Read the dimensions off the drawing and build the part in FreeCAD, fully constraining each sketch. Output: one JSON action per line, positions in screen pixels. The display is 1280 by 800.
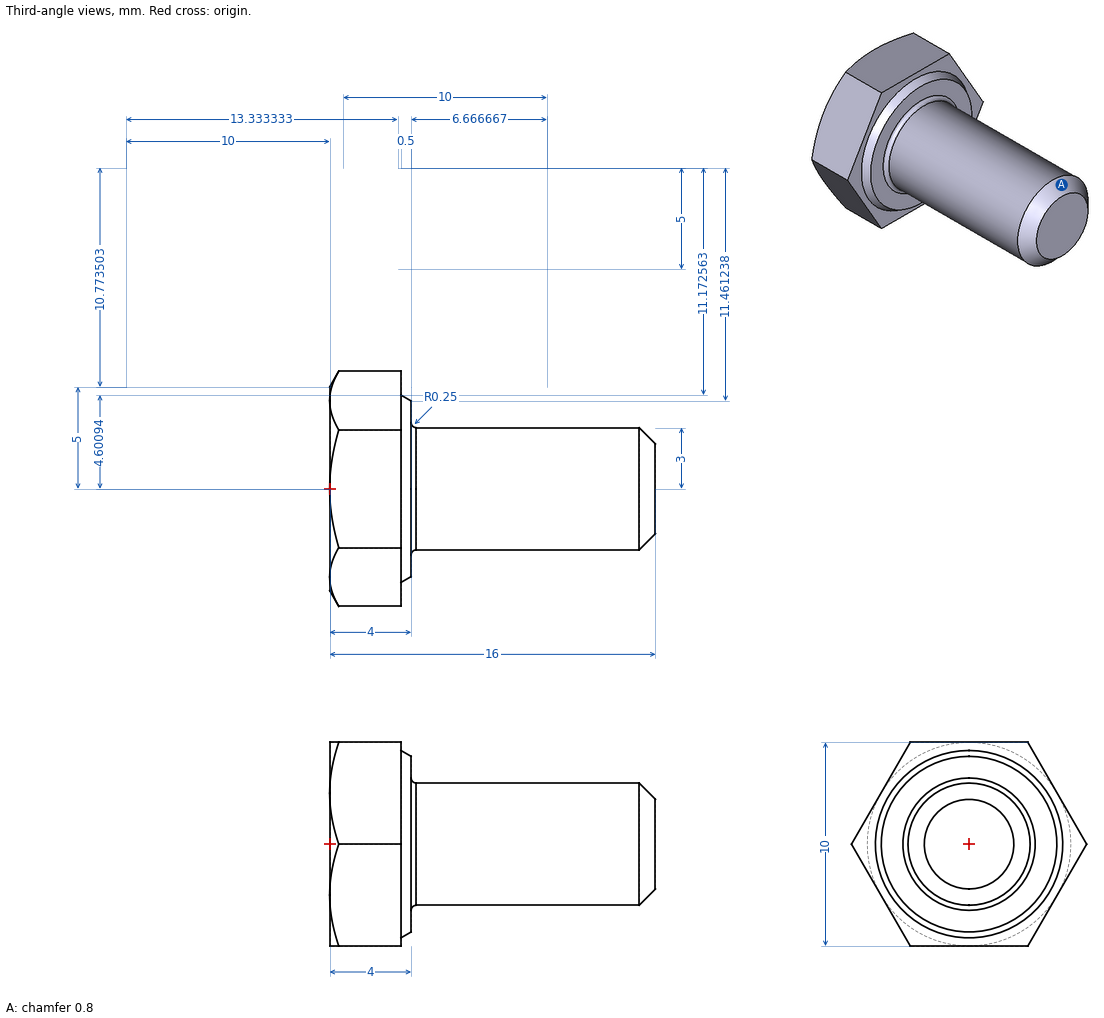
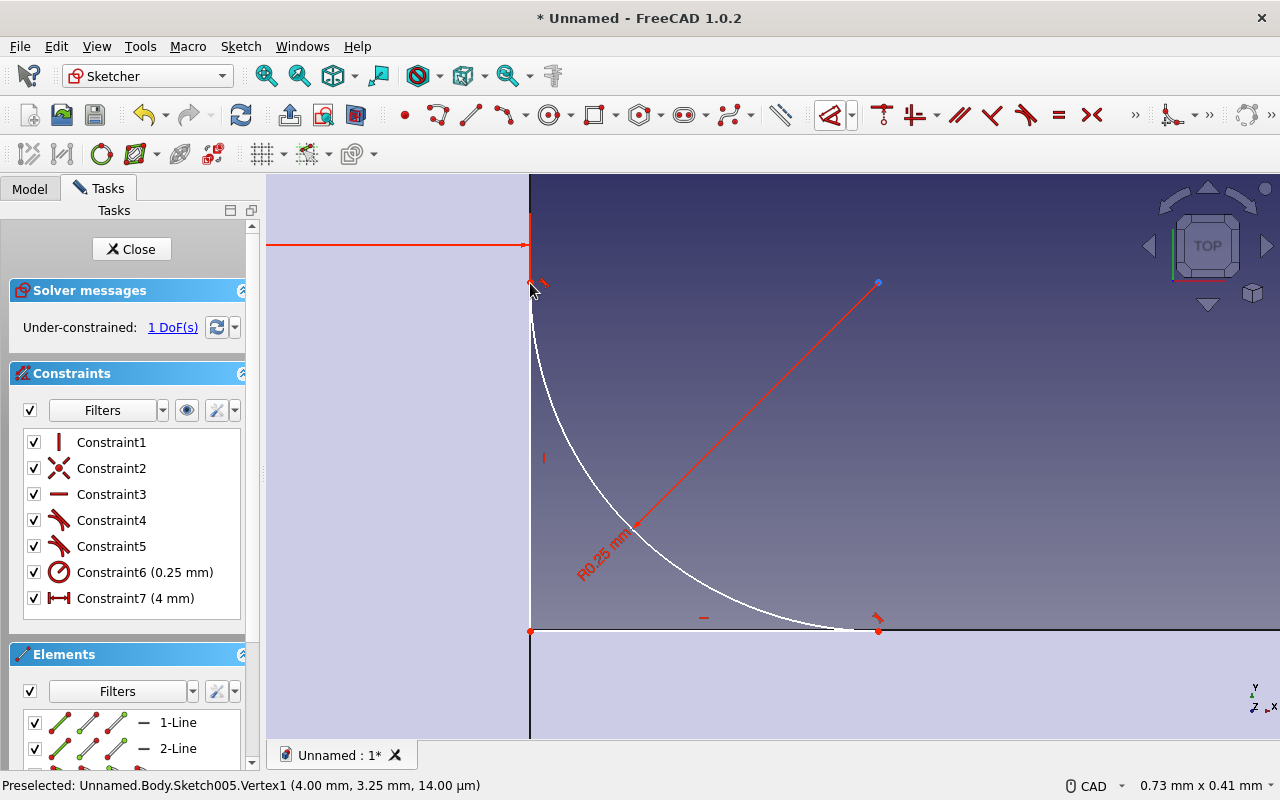
{"action": "left_click", "coordinate": [530, 631]}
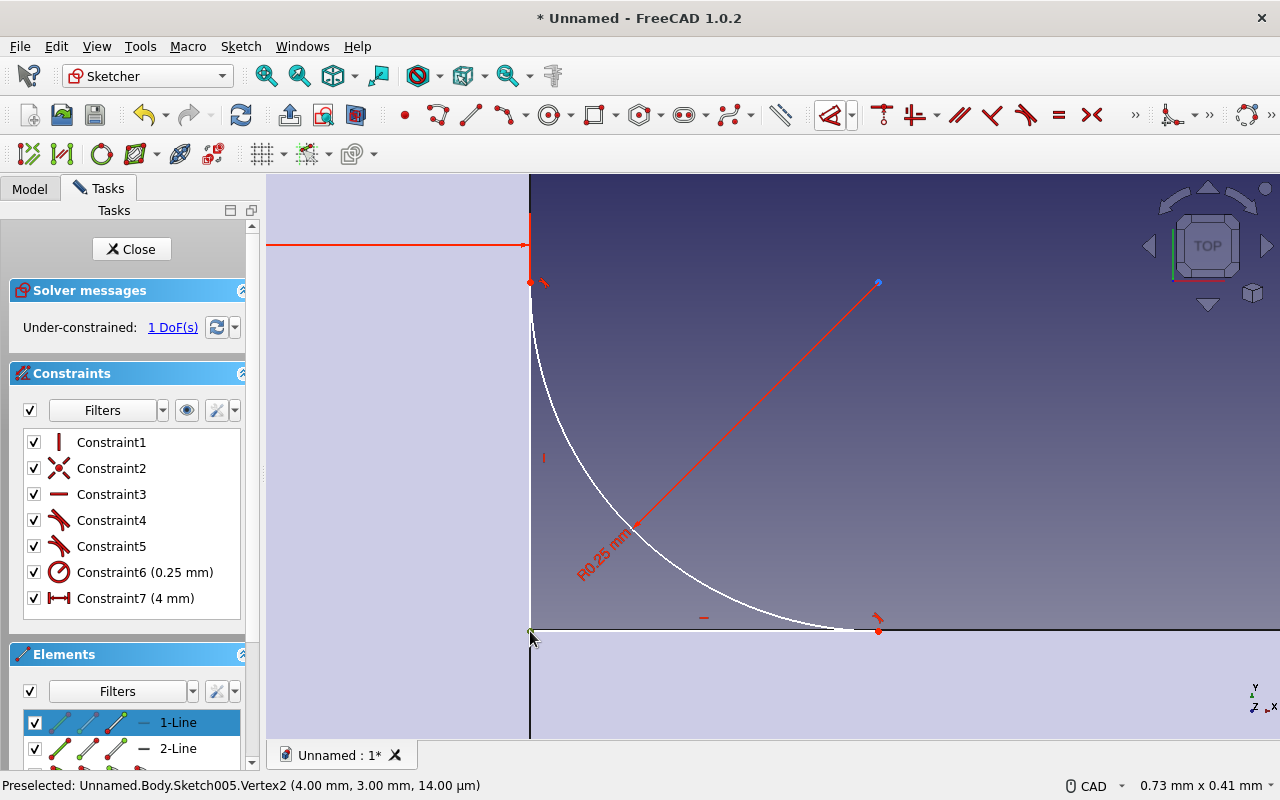
{"action": "left_click", "coordinate": [852, 116]}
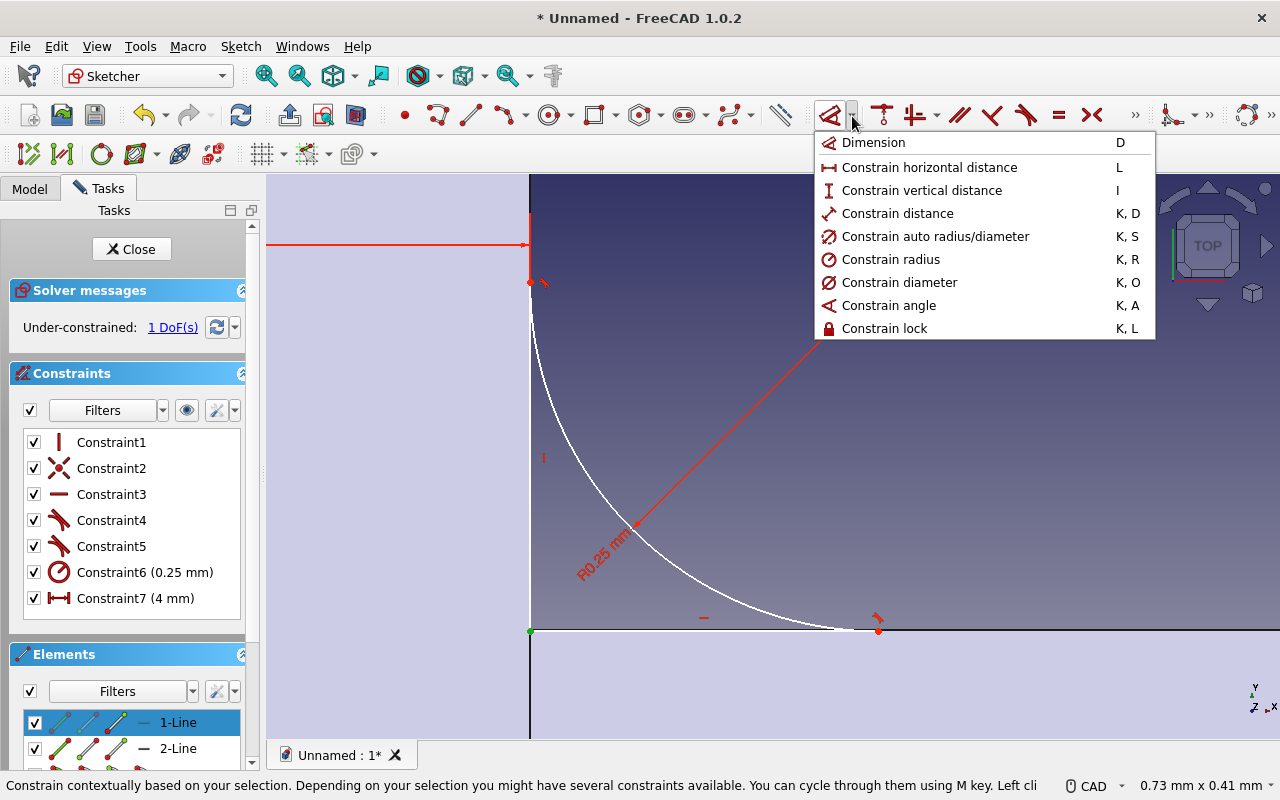
{"action": "left_click", "coordinate": [985, 190]}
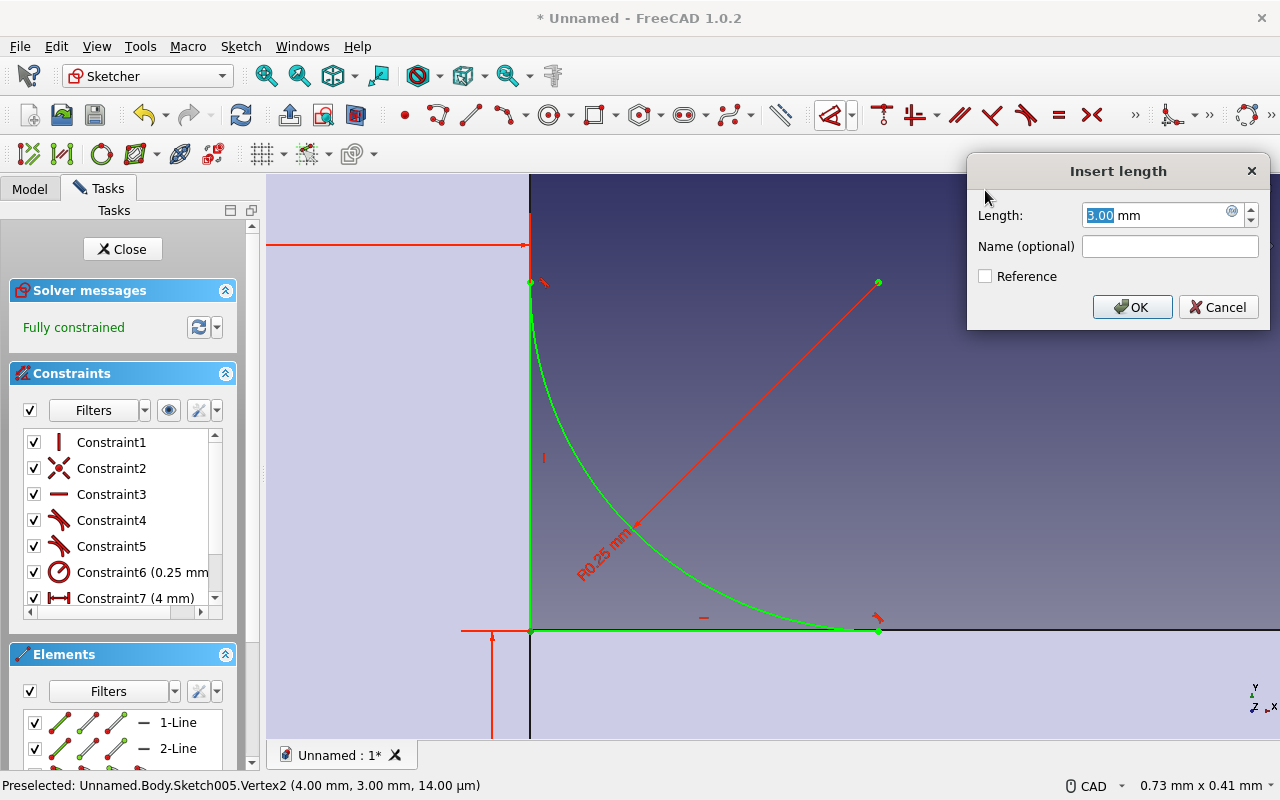
{"action": "type", "text": "3"}
{"action": "key", "text": "Return"}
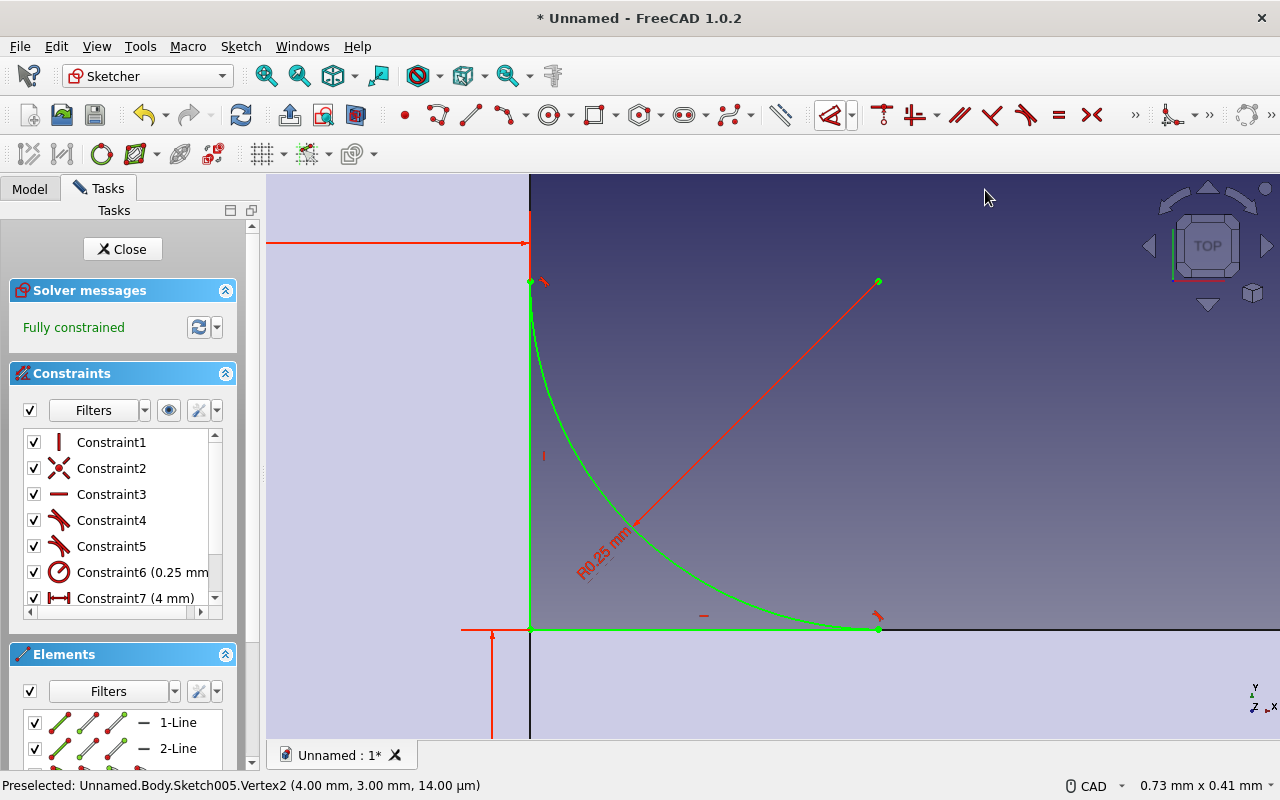
{"action": "left_click", "coordinate": [123, 249]}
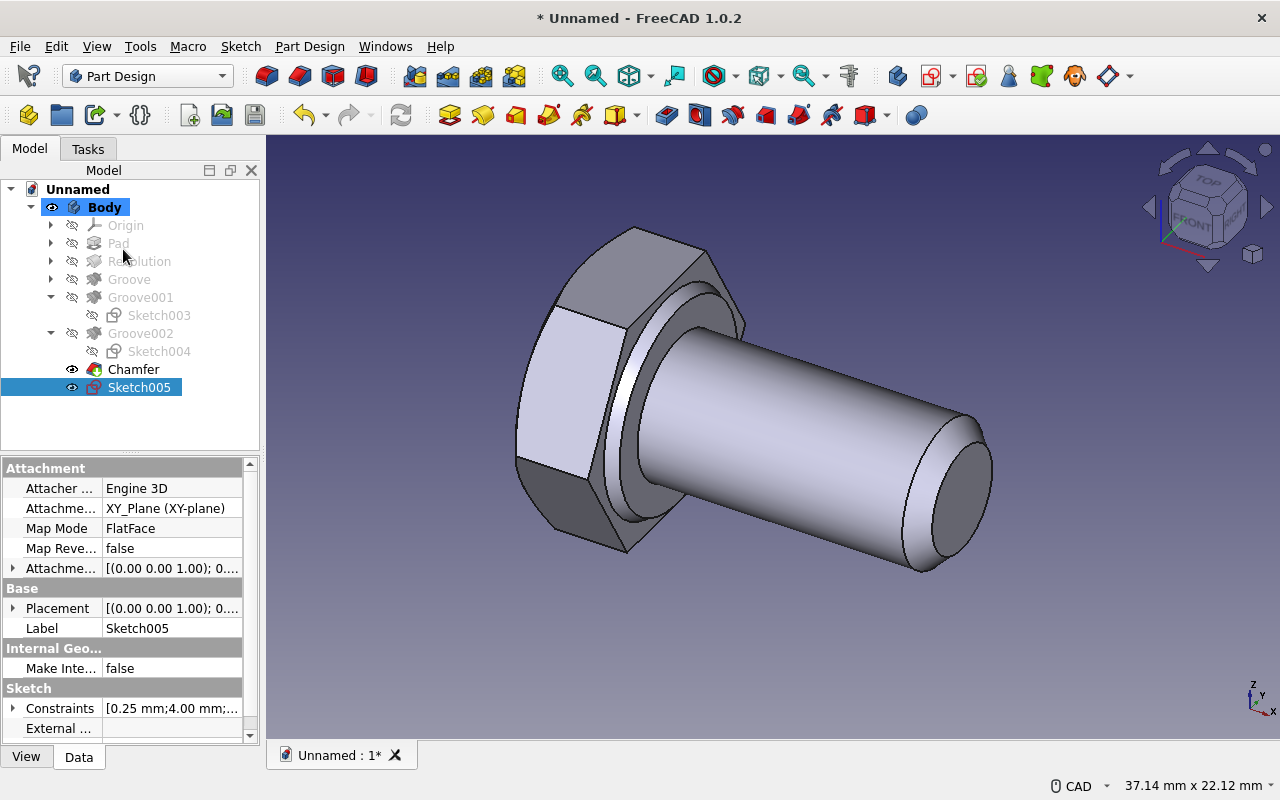
{"action": "left_click", "coordinate": [483, 116]}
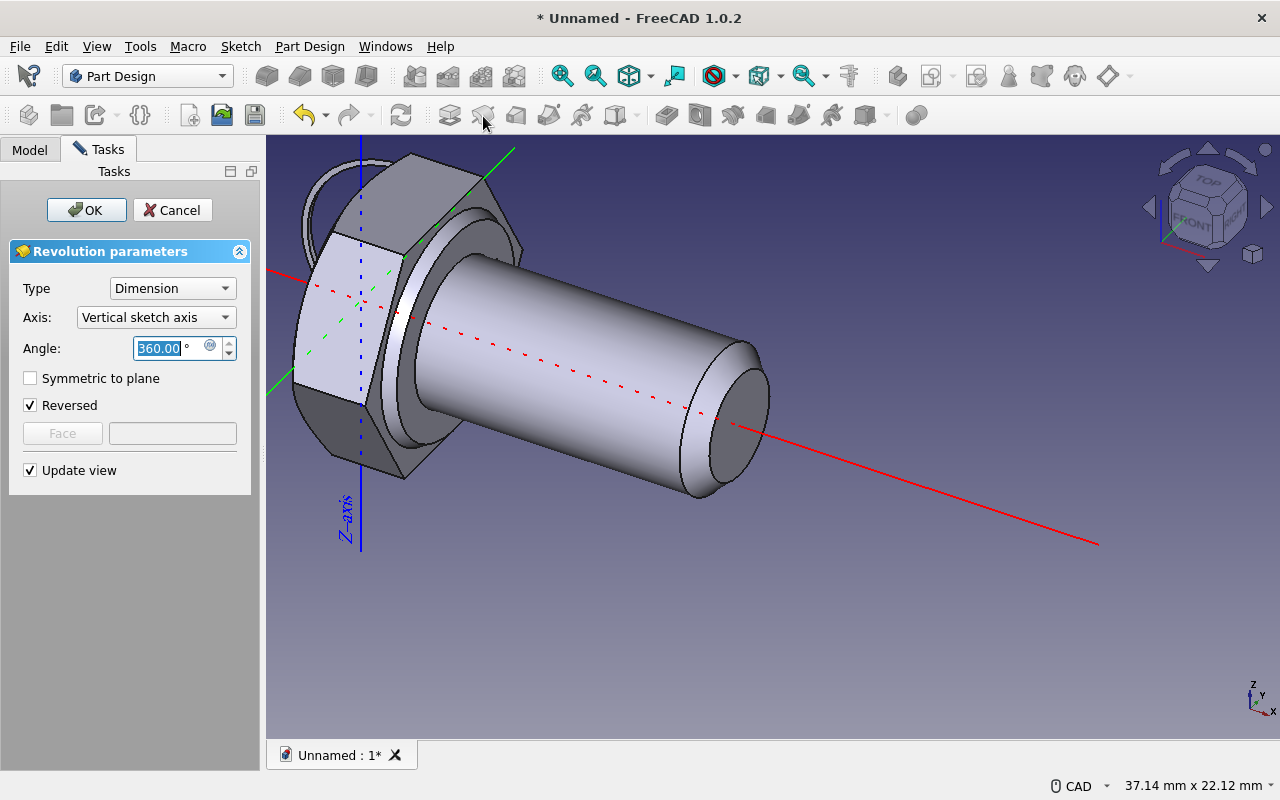
{"action": "left_click", "coordinate": [157, 318]}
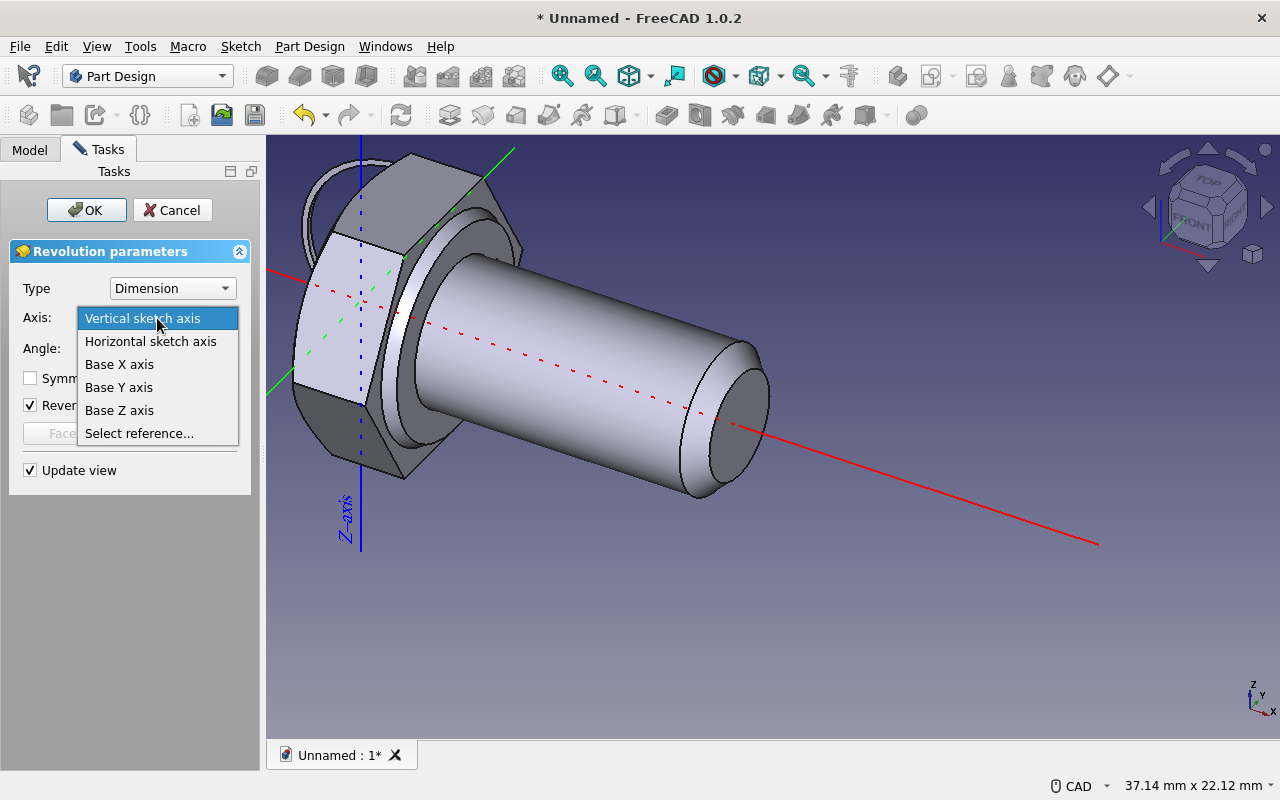
{"action": "left_click", "coordinate": [156, 342]}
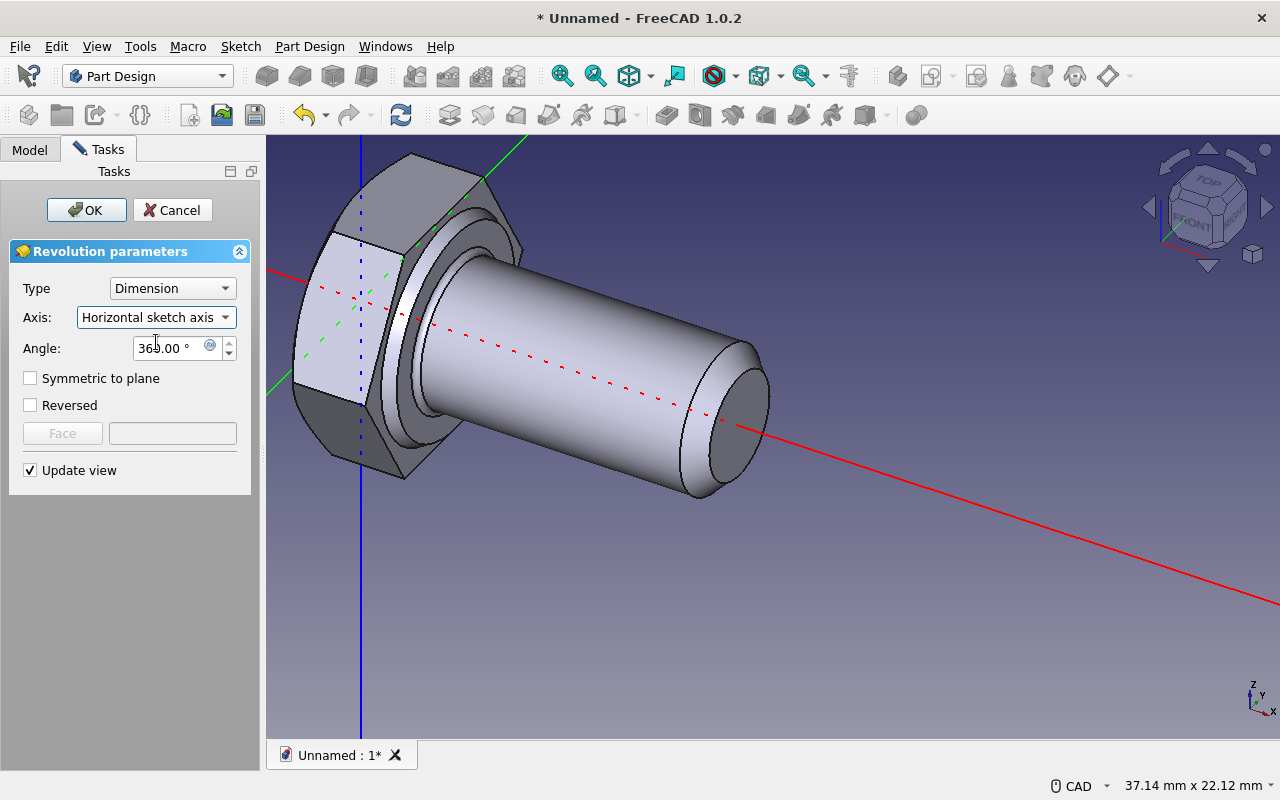
{"action": "left_click", "coordinate": [87, 210]}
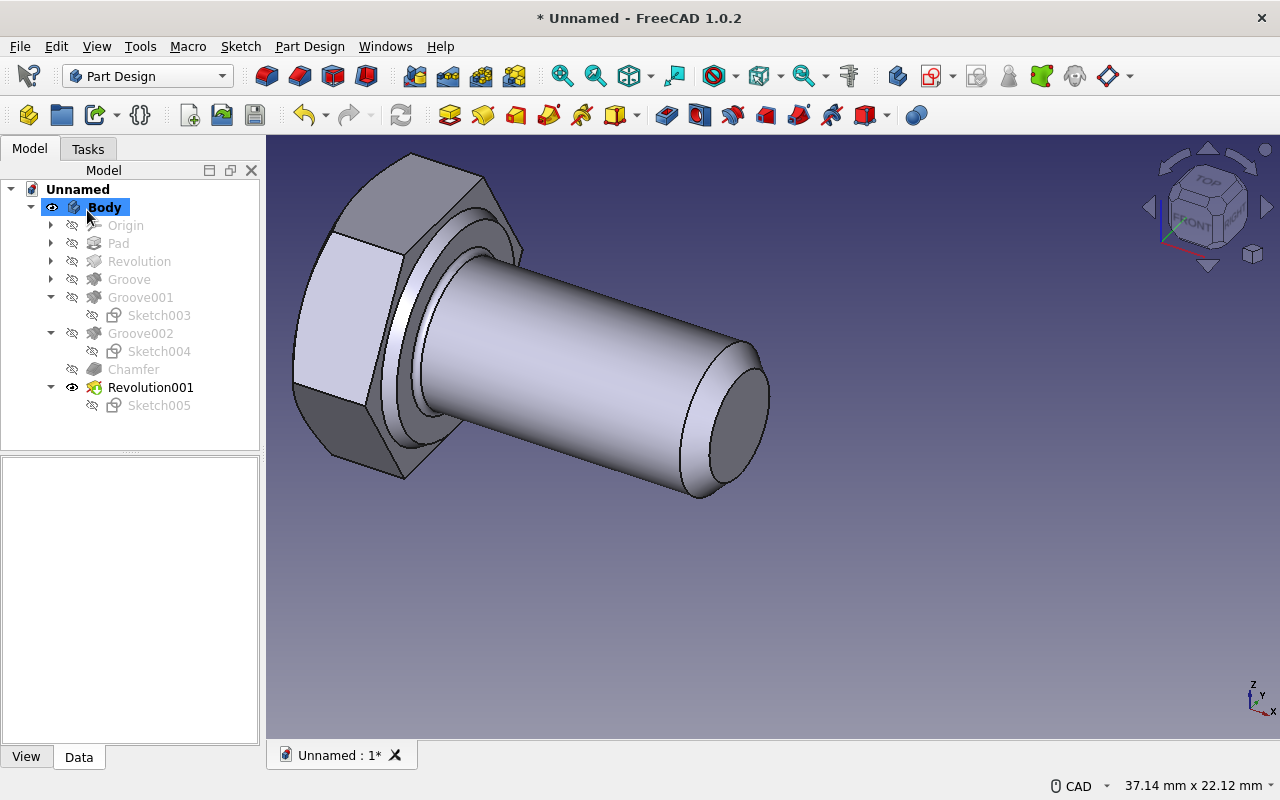
{"action": "key", "text": "0"}